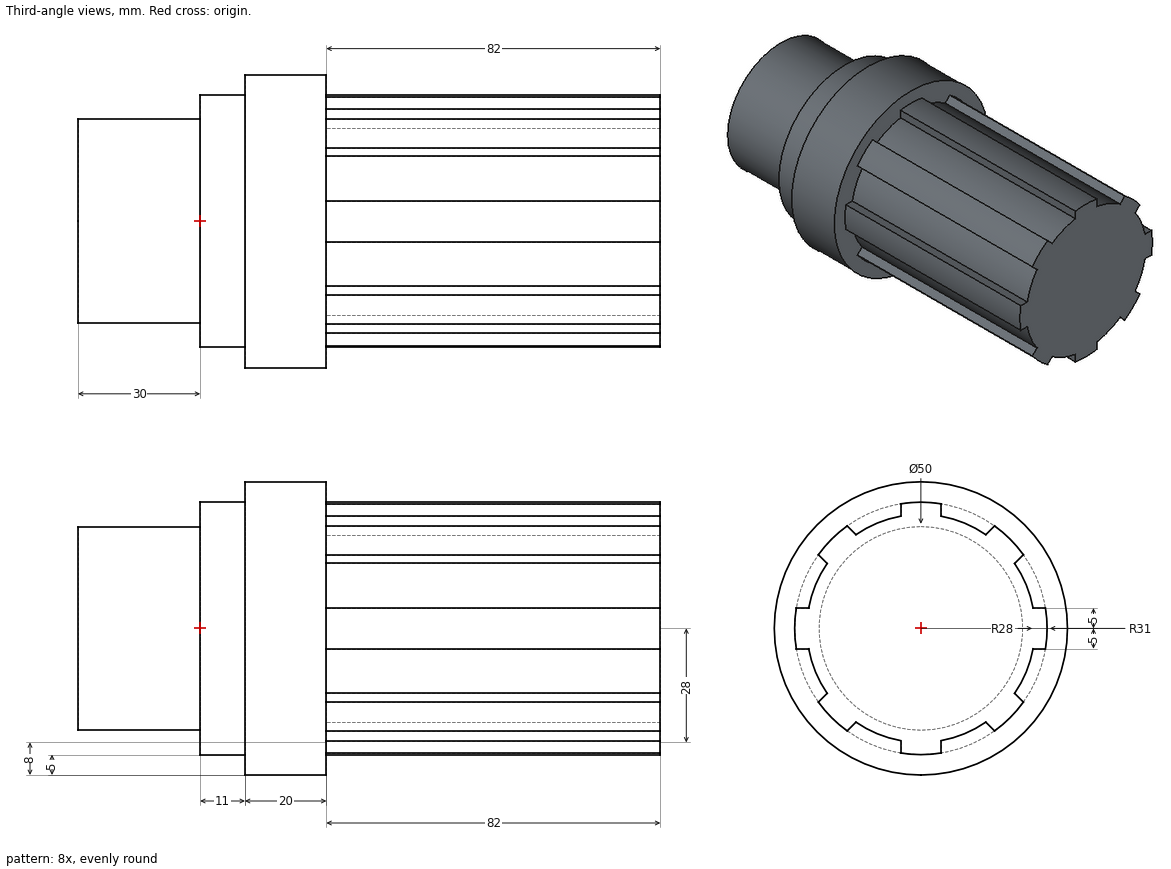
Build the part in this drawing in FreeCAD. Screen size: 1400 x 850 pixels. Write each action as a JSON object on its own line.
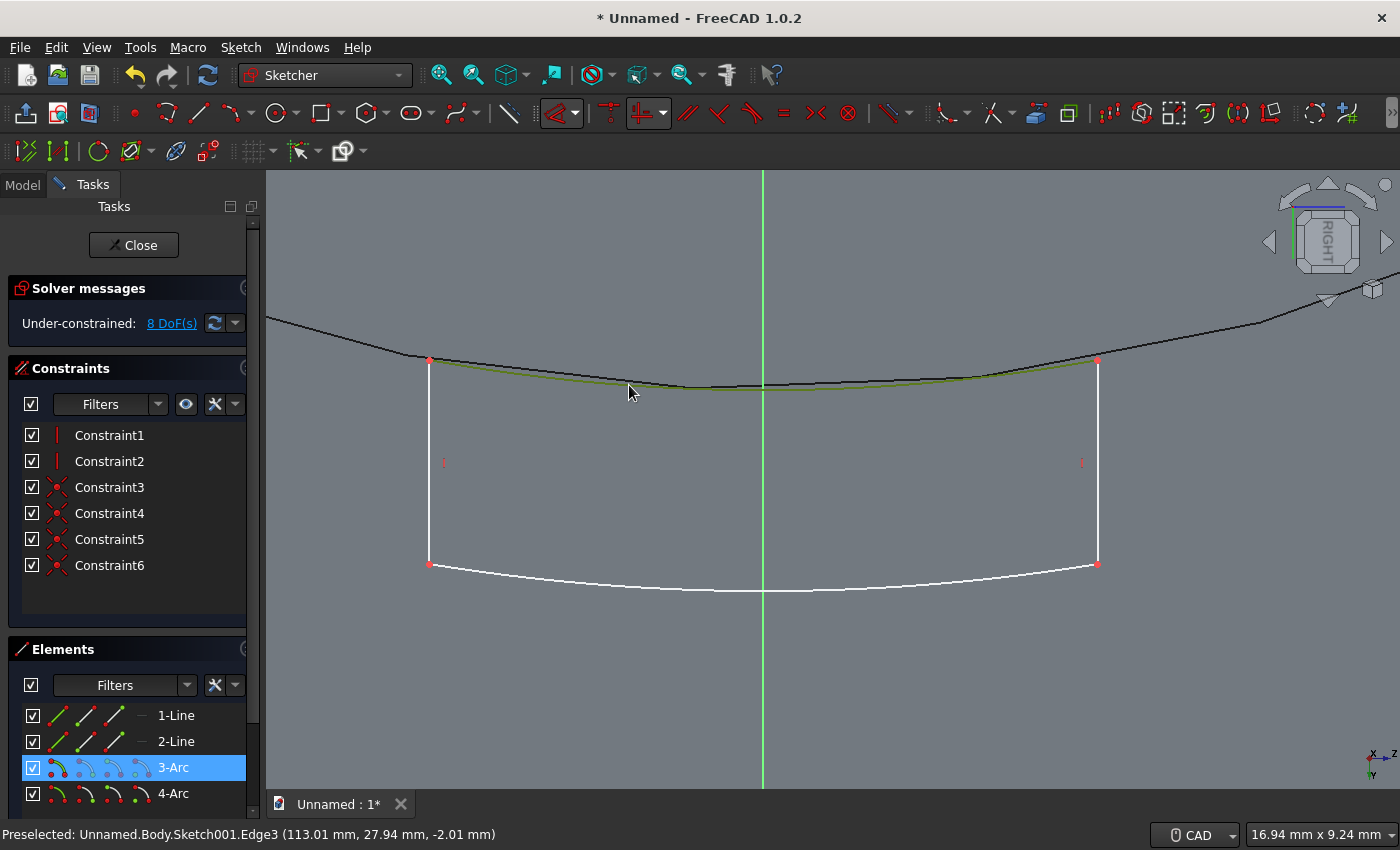
{"action": "left_click", "coordinate": [629, 587]}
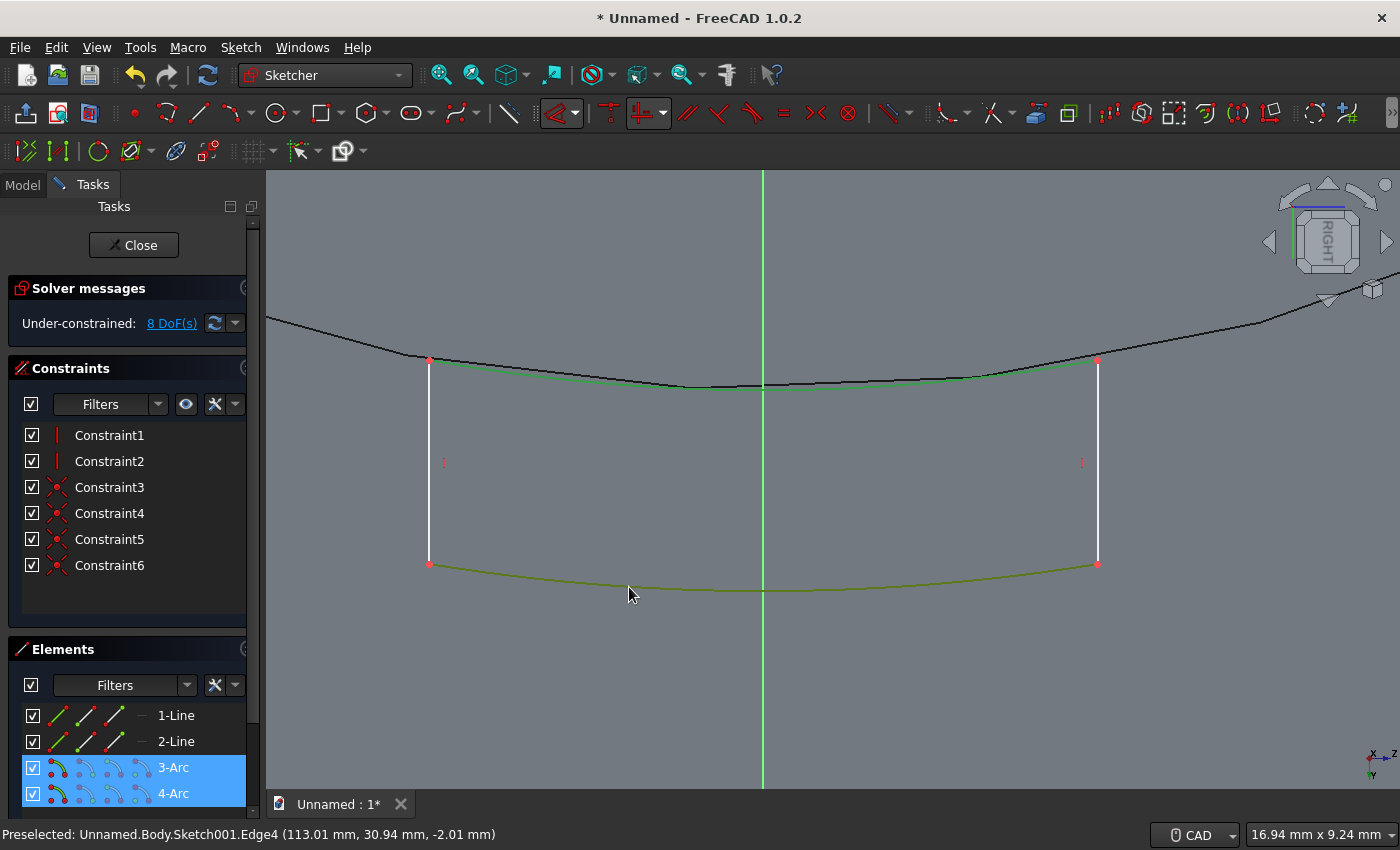
{"action": "left_click", "coordinate": [610, 114]}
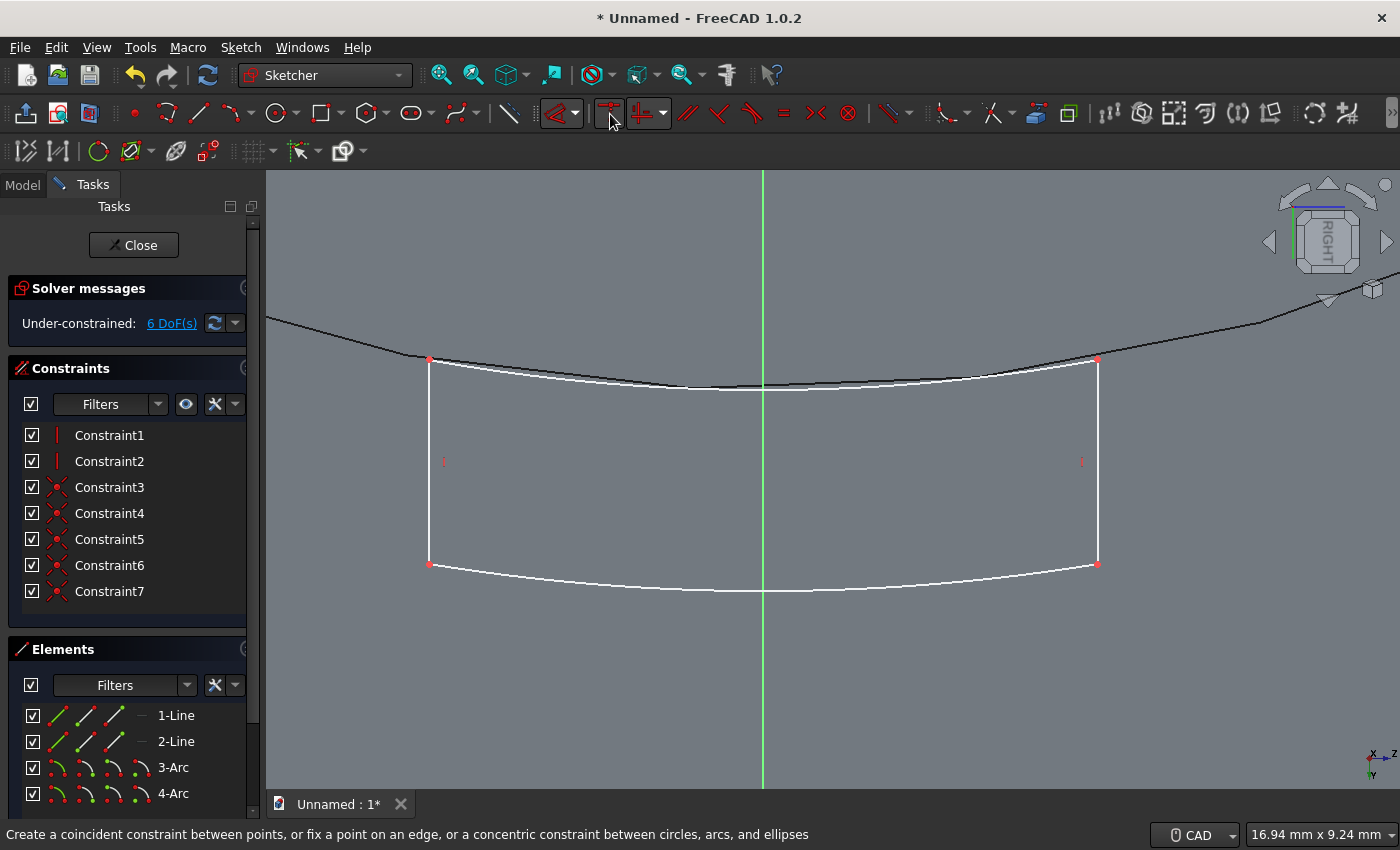
{"action": "scroll", "coordinate": [765, 714], "scroll_direction": "down", "scroll_amount": 8}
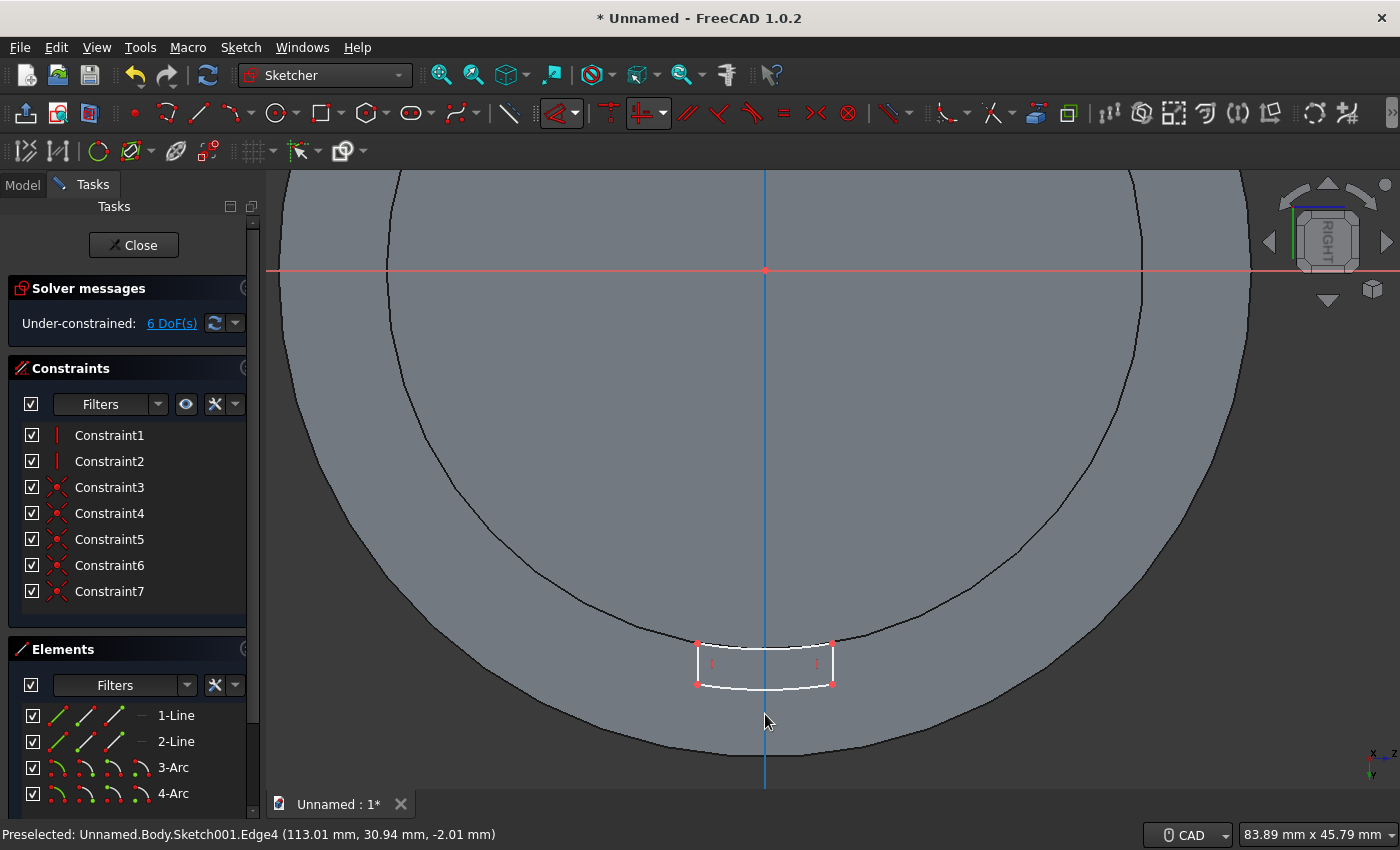
{"action": "left_click_drag", "start_coordinate": [755, 260], "coordinate": [775, 281]}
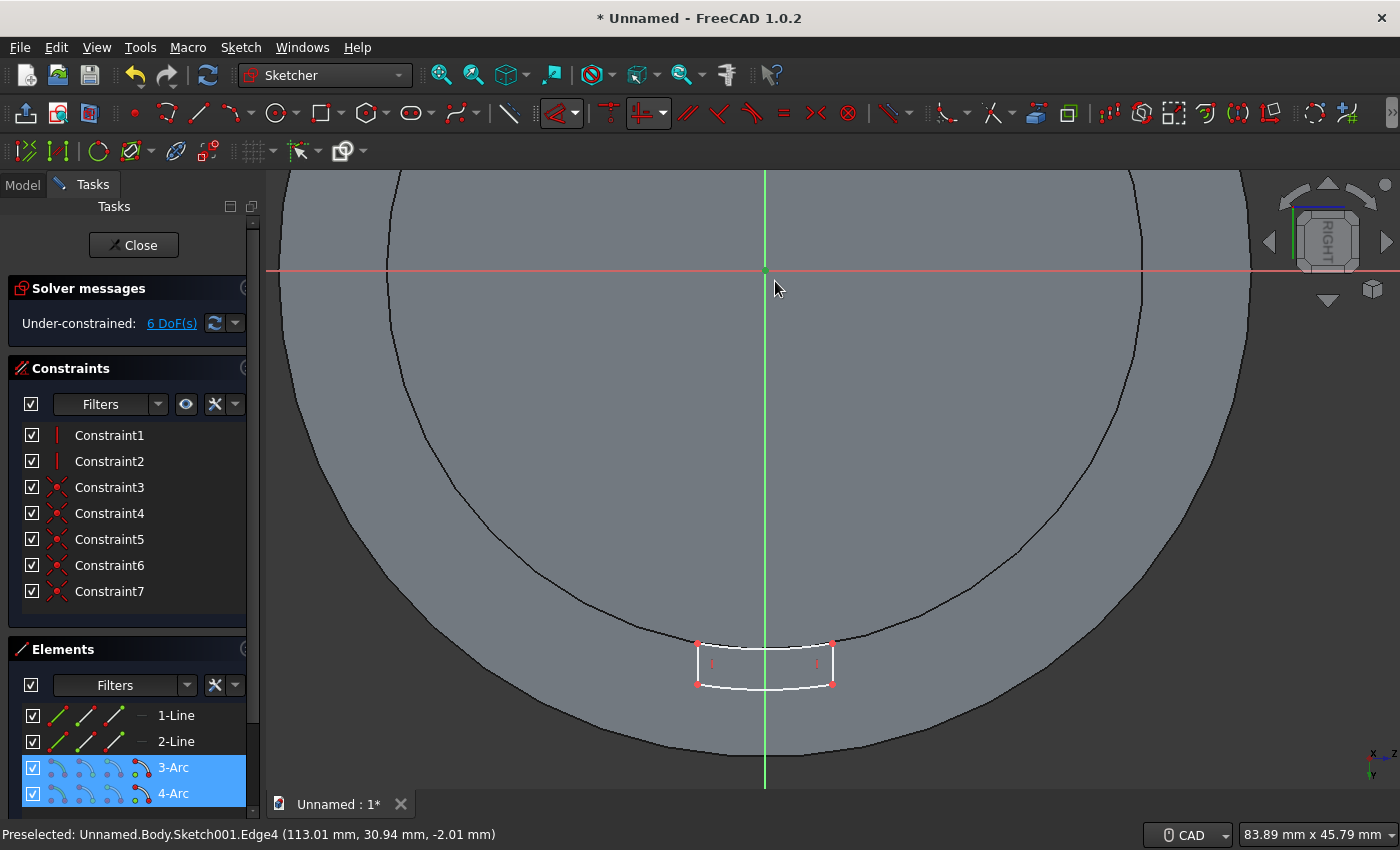
{"action": "left_click", "coordinate": [610, 114]}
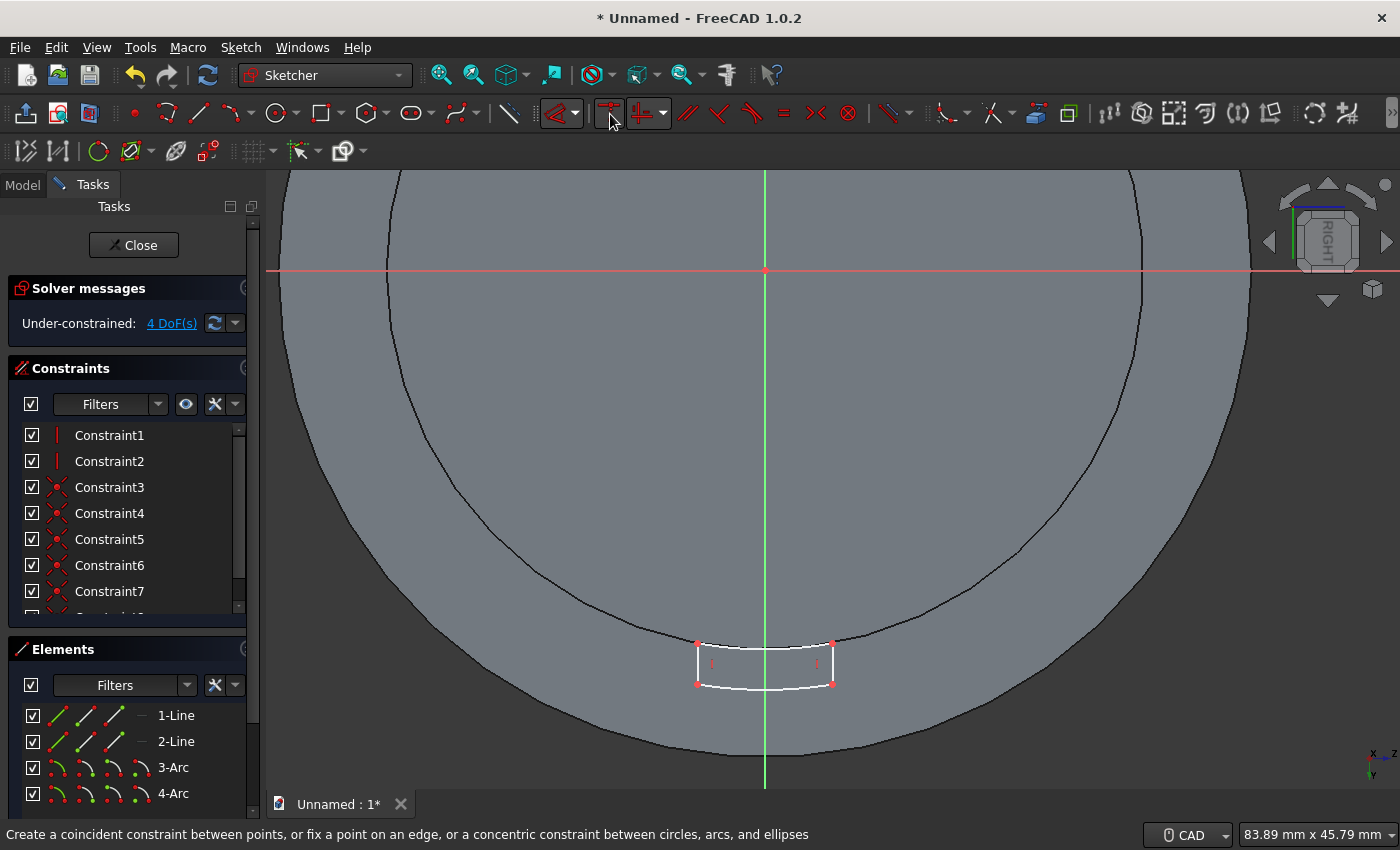
{"action": "left_click", "coordinate": [738, 648]}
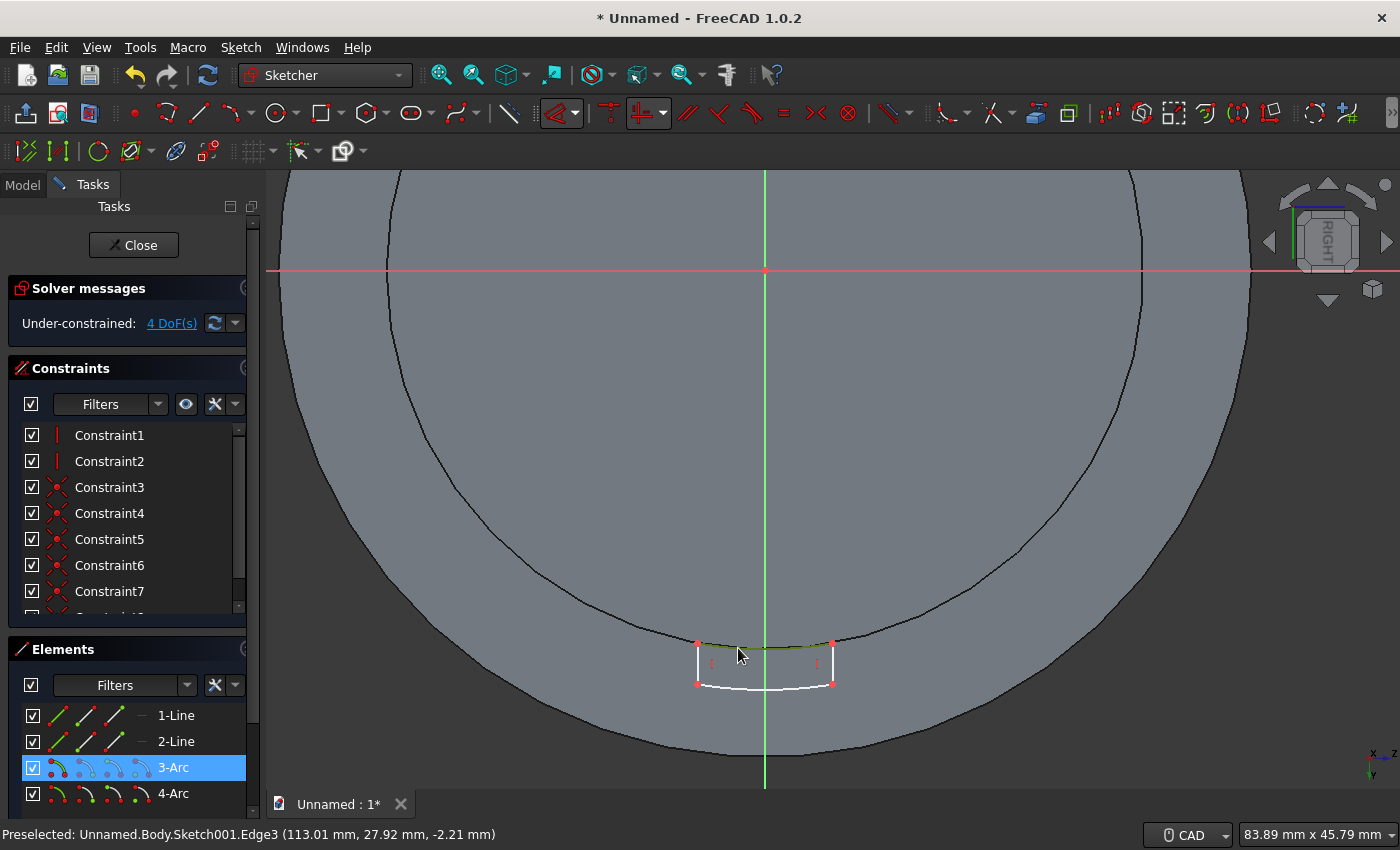
{"action": "left_click", "coordinate": [578, 114]}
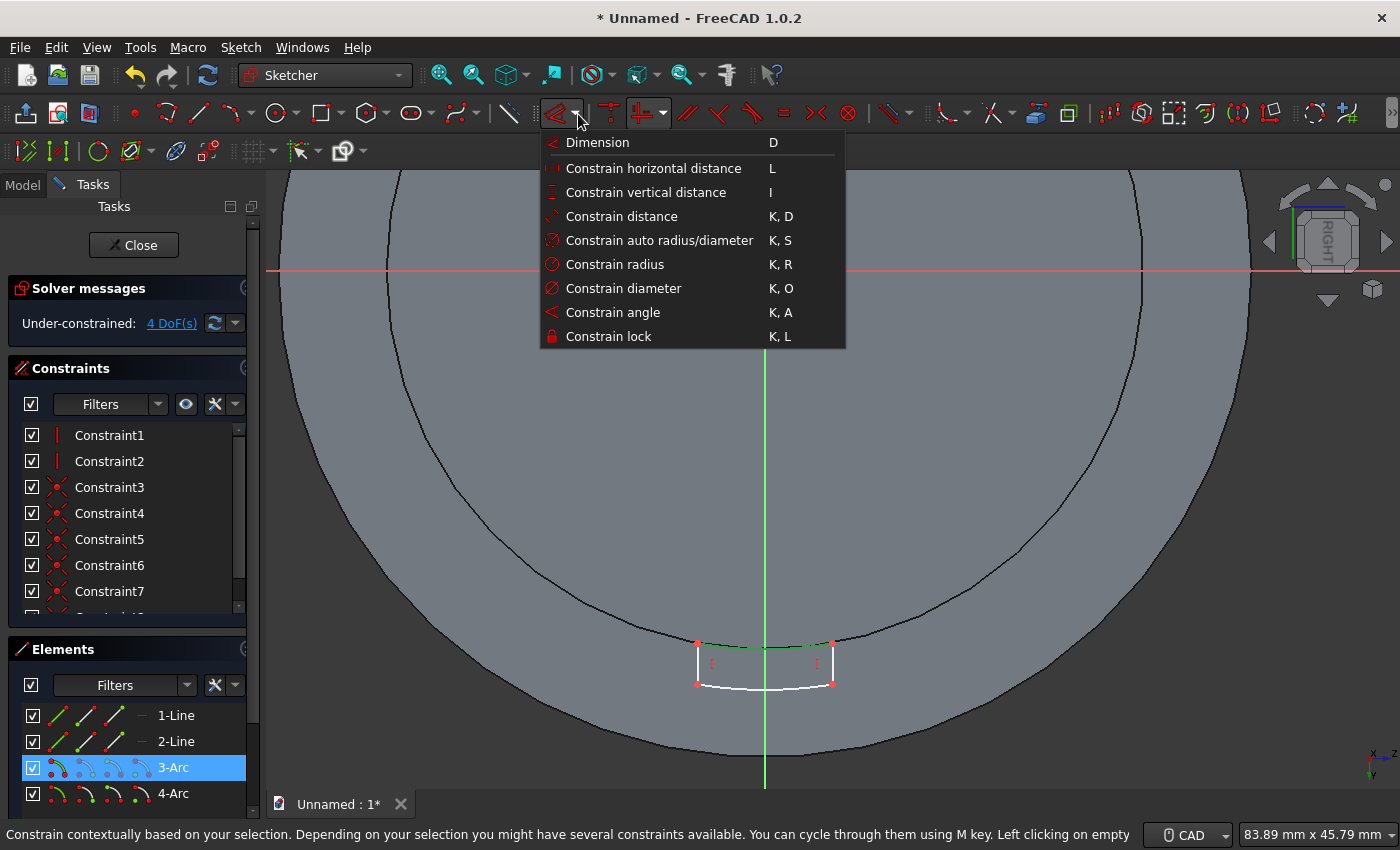
{"action": "left_click", "coordinate": [693, 264]}